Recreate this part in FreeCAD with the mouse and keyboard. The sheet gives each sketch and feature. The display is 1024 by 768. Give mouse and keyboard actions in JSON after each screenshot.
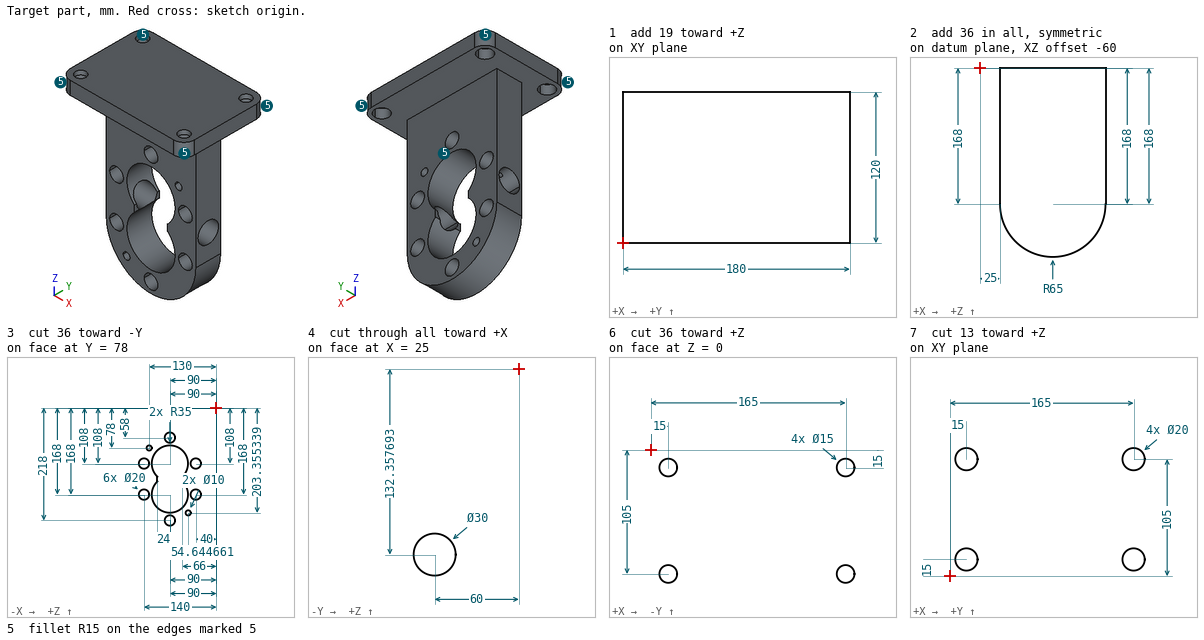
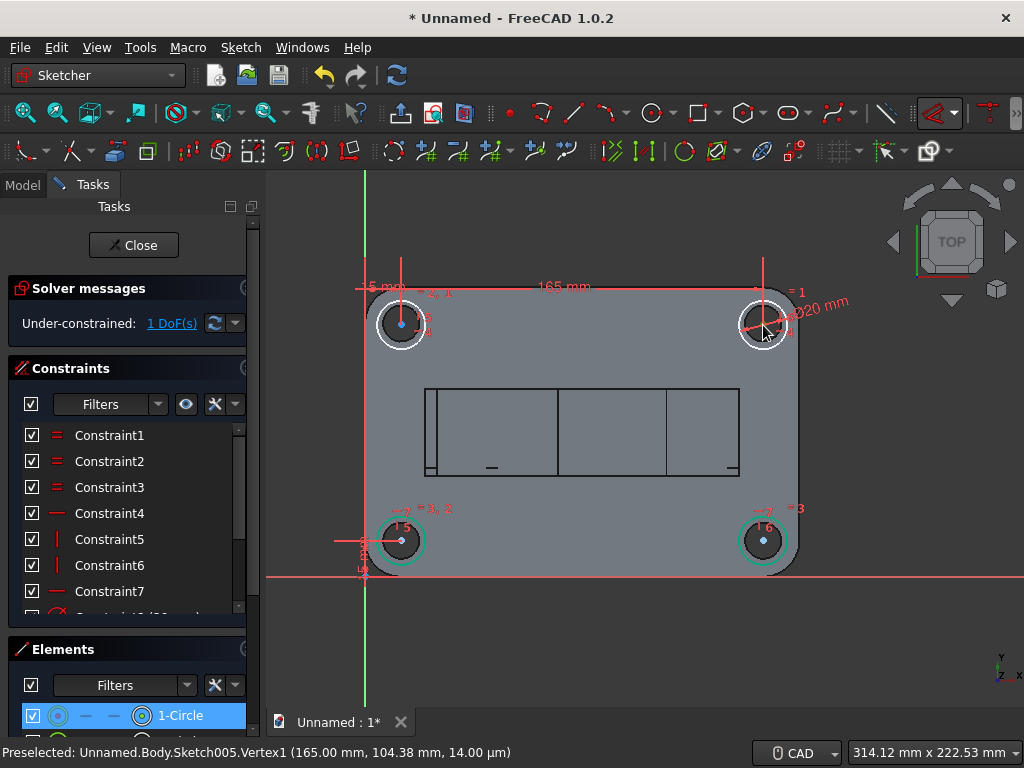
{"action": "left_click", "coordinate": [956, 114]}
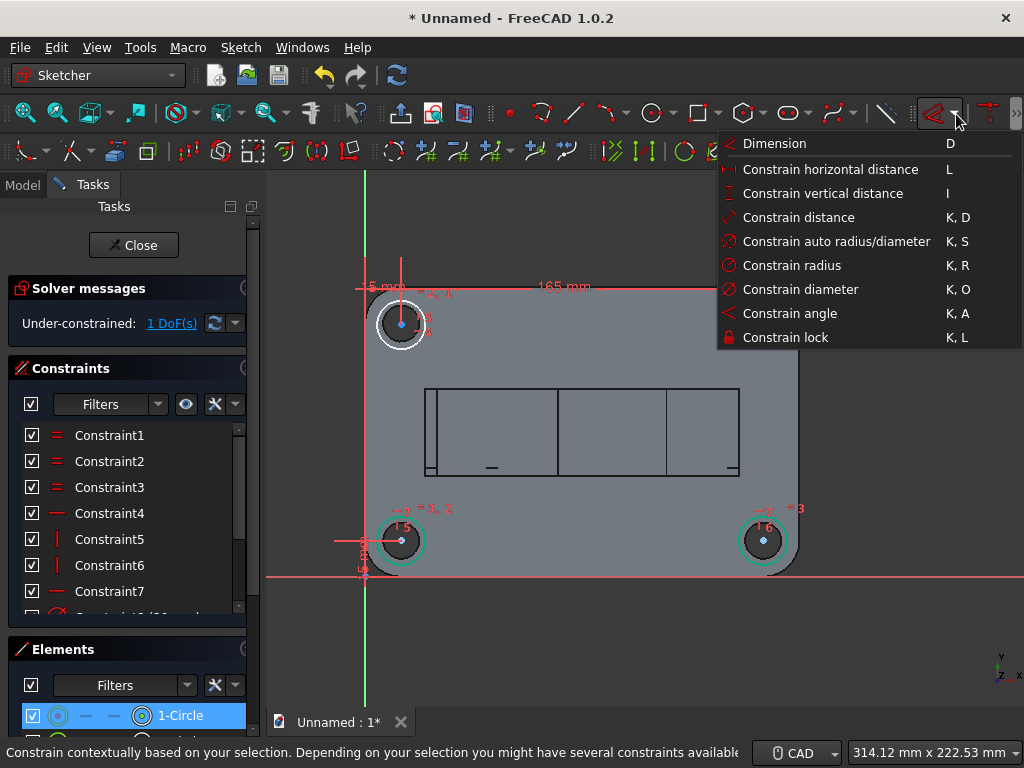
{"action": "left_click", "coordinate": [870, 193]}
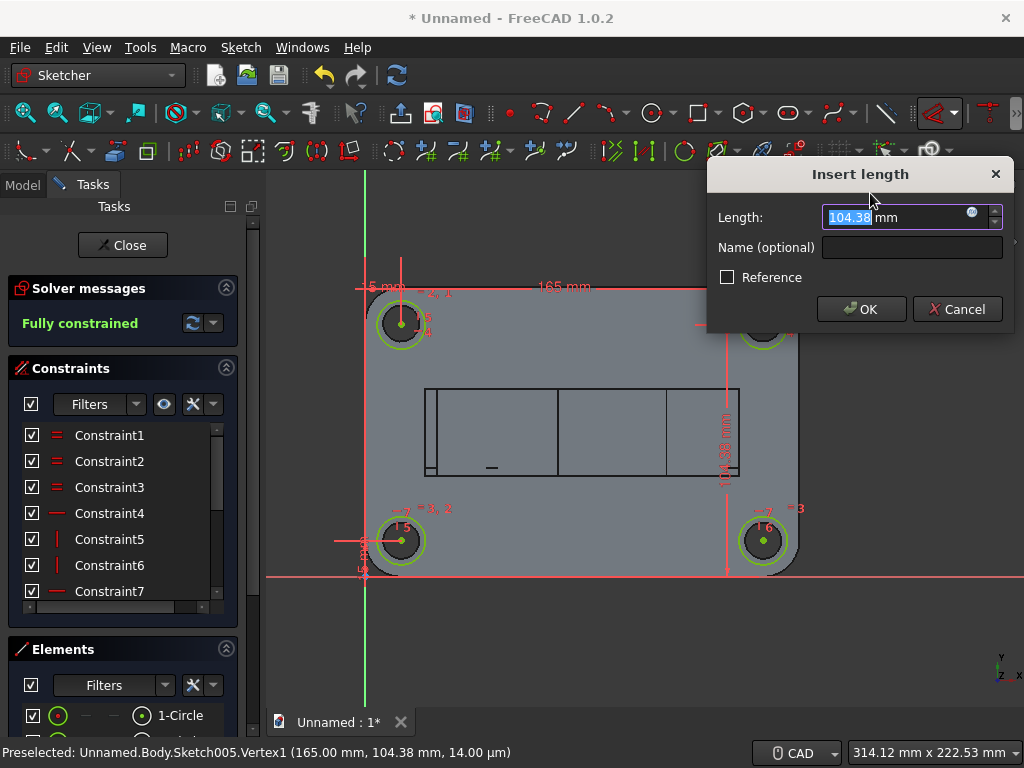
{"action": "type", "text": "105"}
{"action": "key", "text": "Return"}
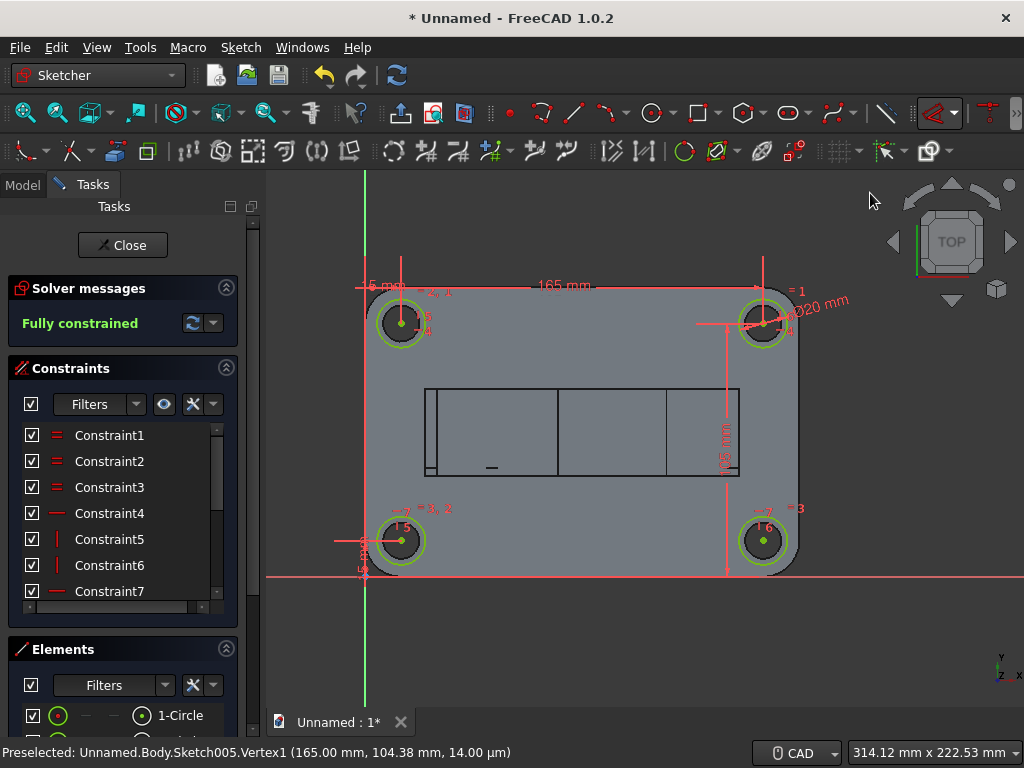
{"action": "left_click", "coordinate": [123, 245]}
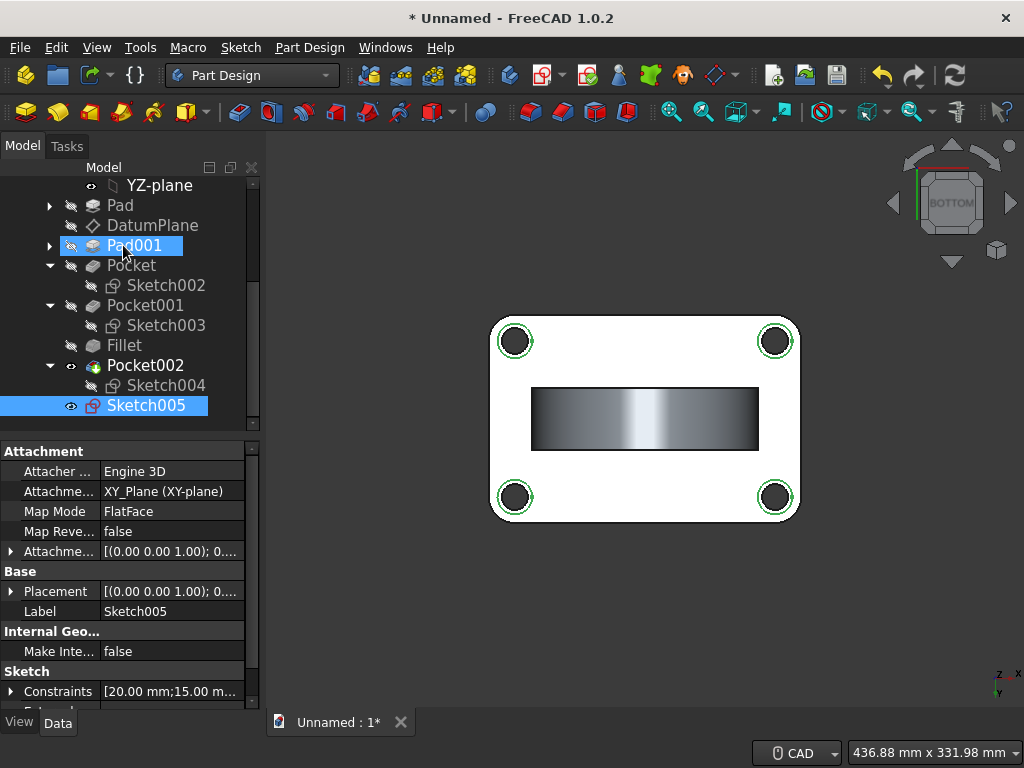
{"action": "left_click", "coordinate": [240, 112]}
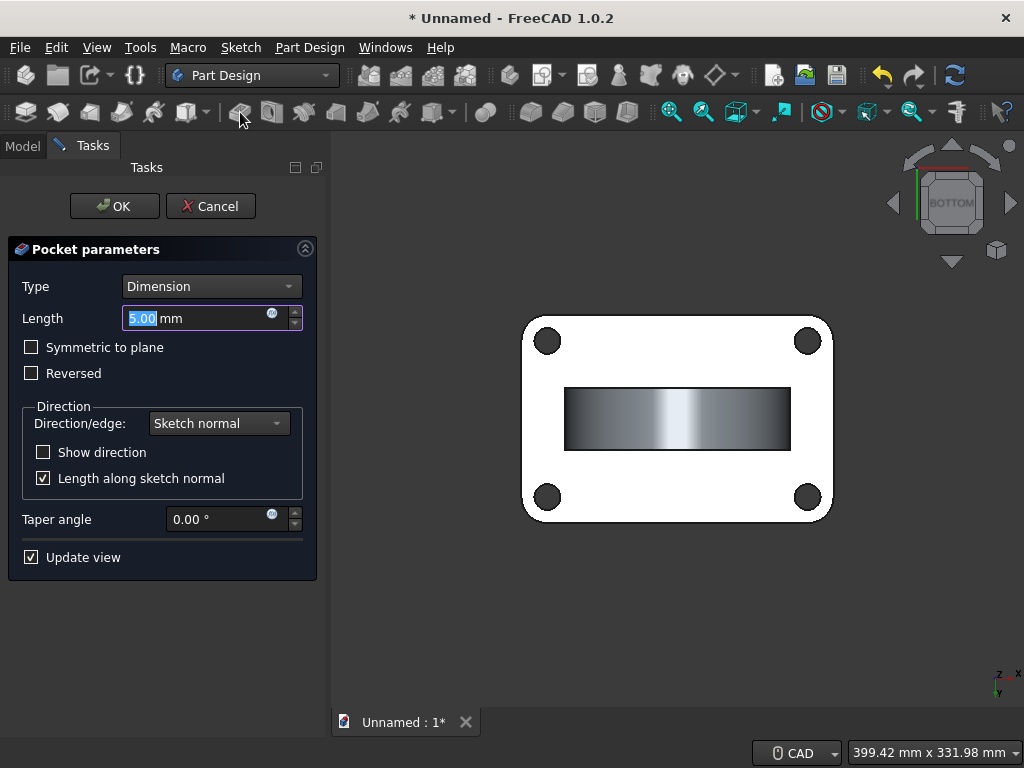
{"action": "type", "text": "13"}
{"action": "key", "text": "Tab"}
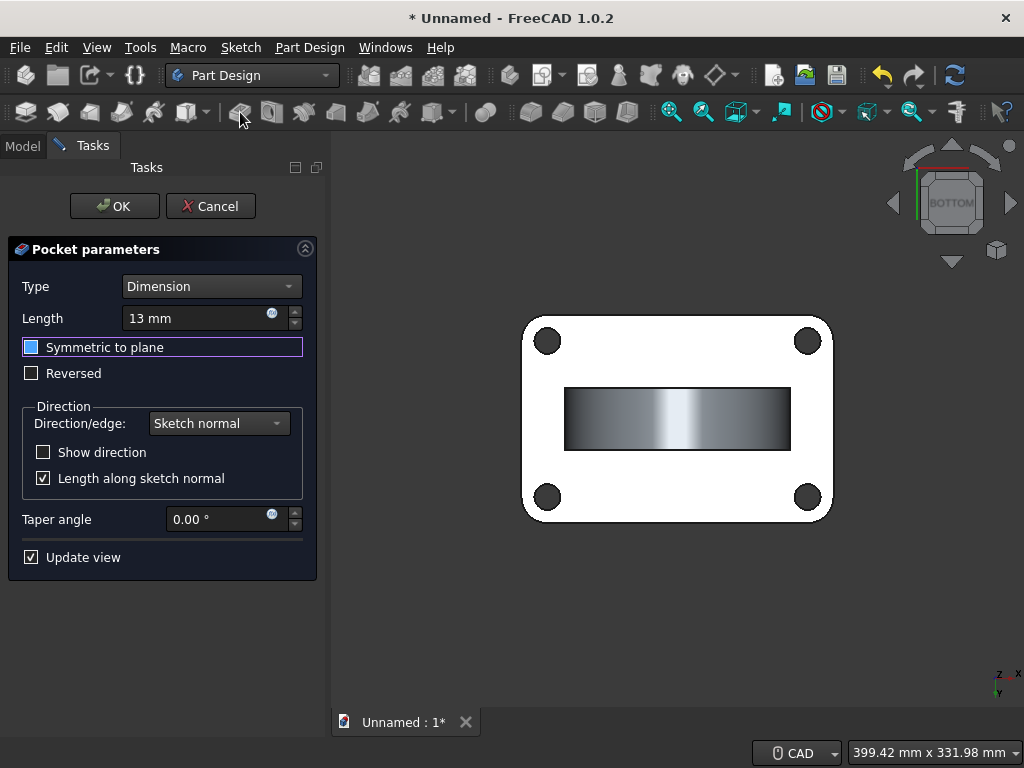
{"action": "left_click", "coordinate": [30, 373]}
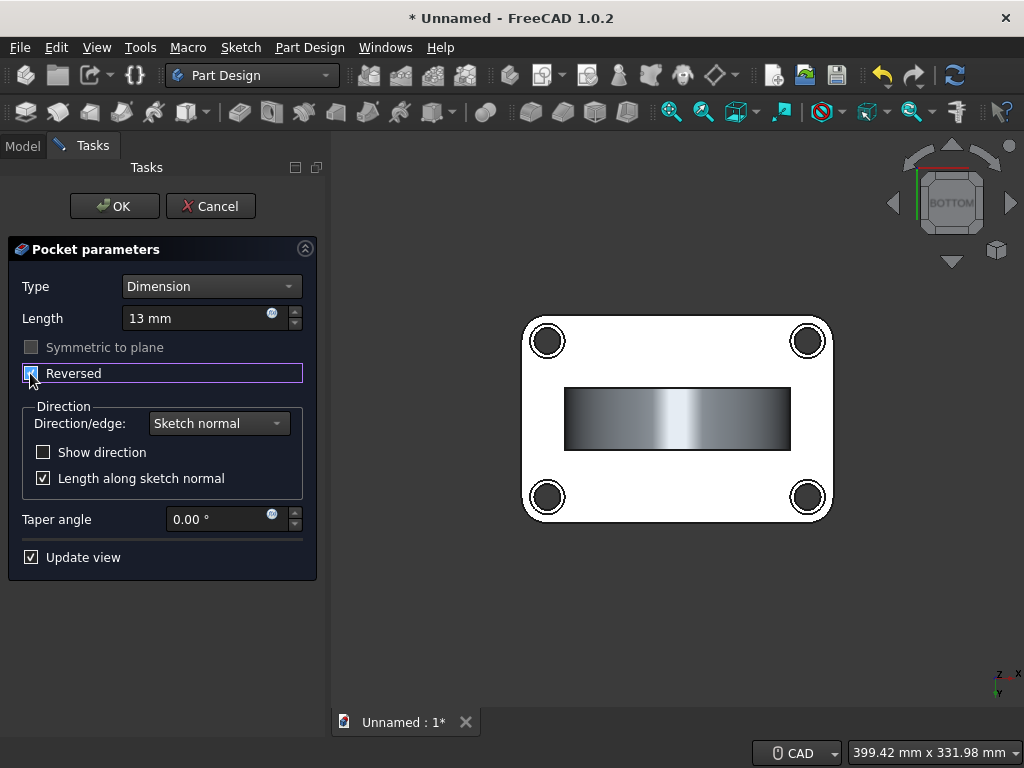
{"action": "left_click", "coordinate": [115, 206]}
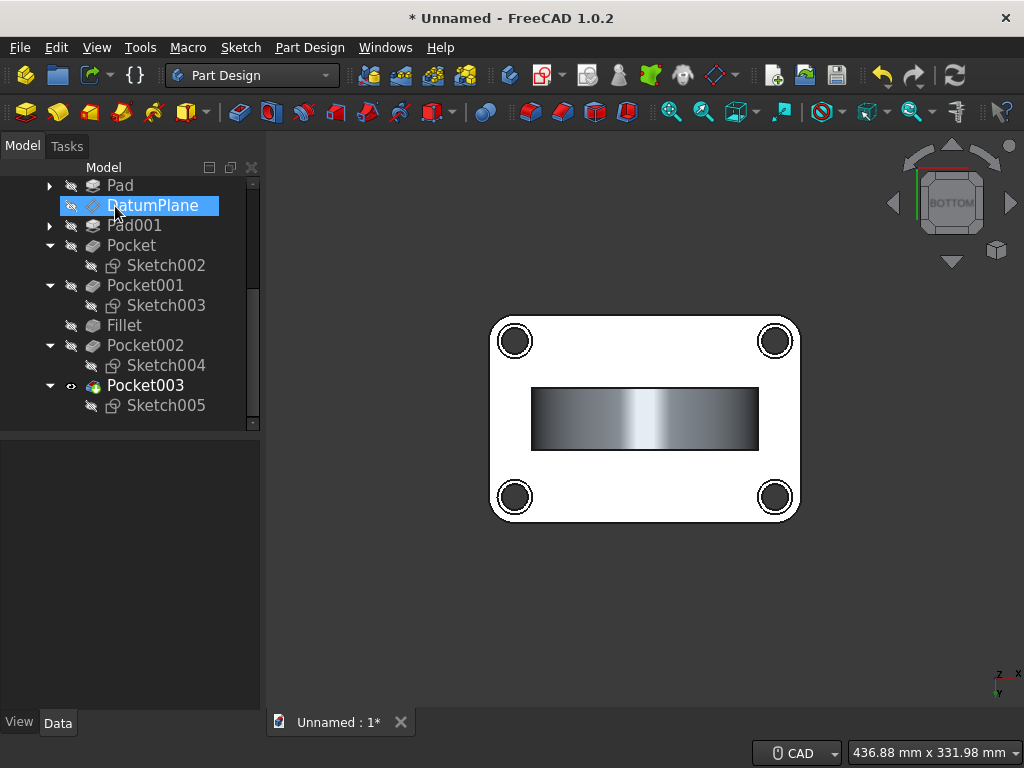
{"action": "key", "text": "0"}